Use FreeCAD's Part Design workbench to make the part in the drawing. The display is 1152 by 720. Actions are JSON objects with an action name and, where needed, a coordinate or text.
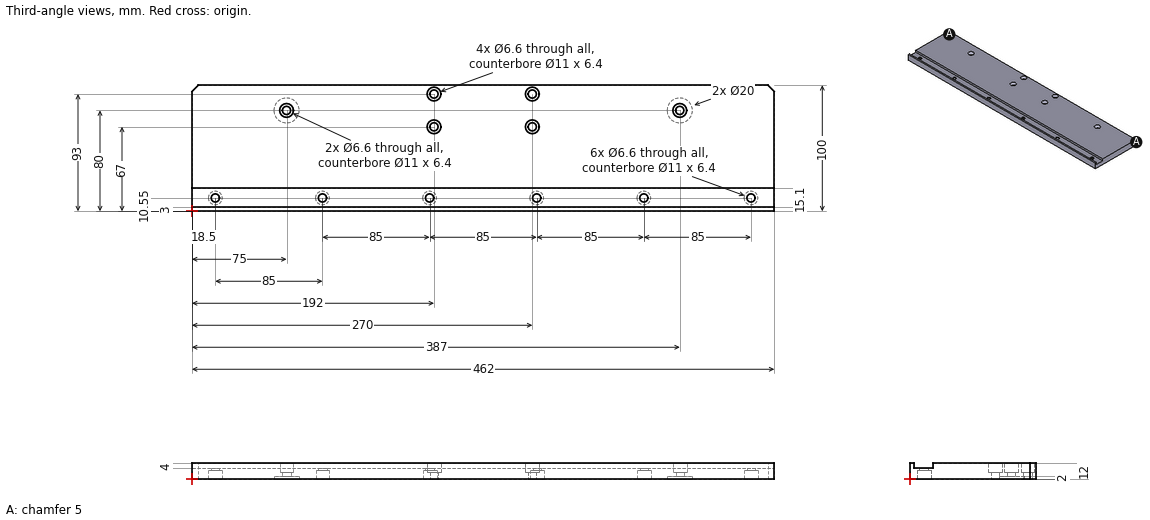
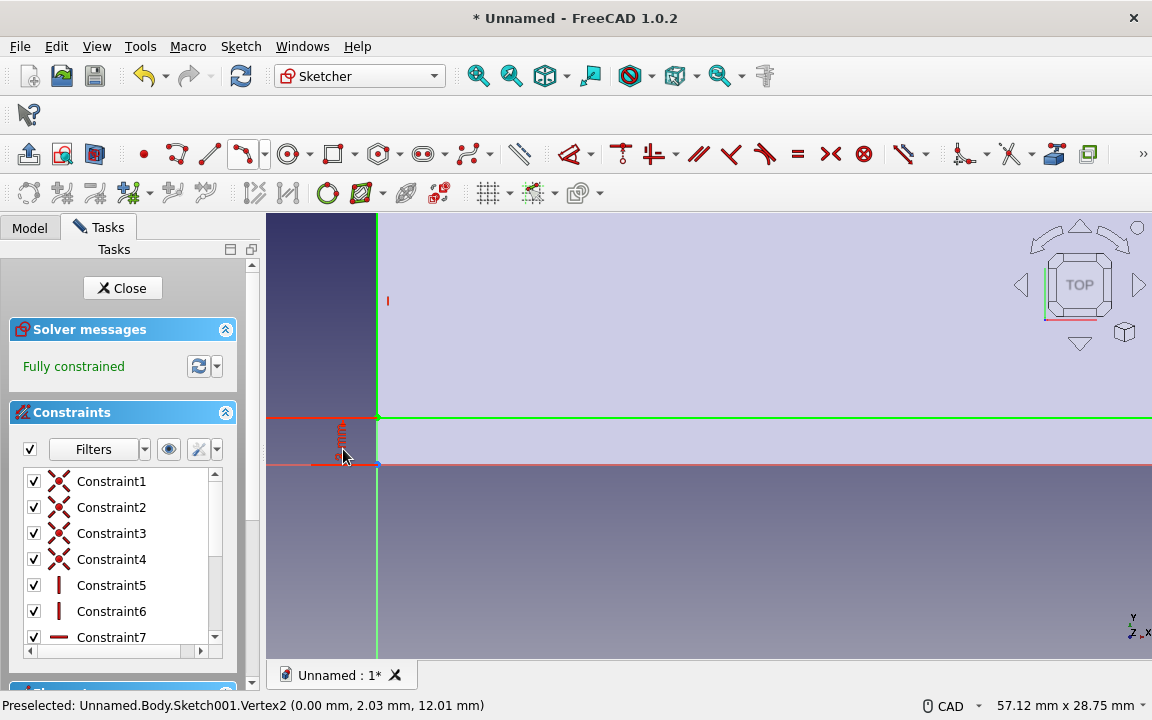
{"action": "left_click", "coordinate": [123, 288]}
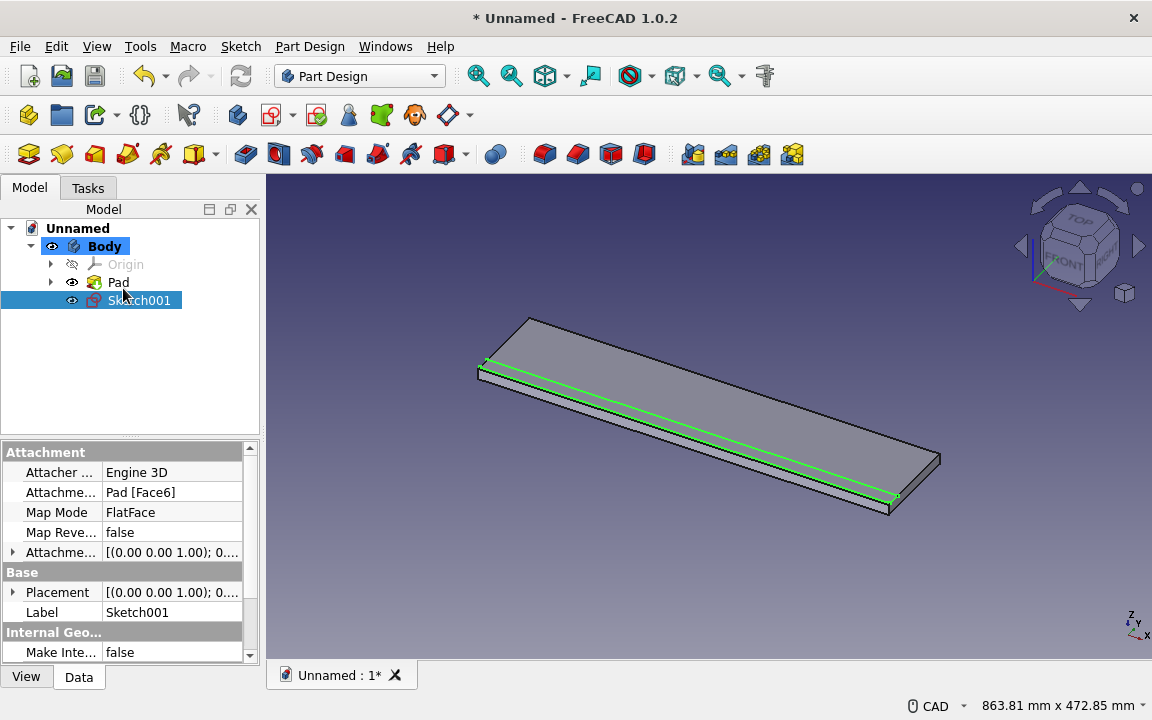
{"action": "left_click", "coordinate": [246, 154]}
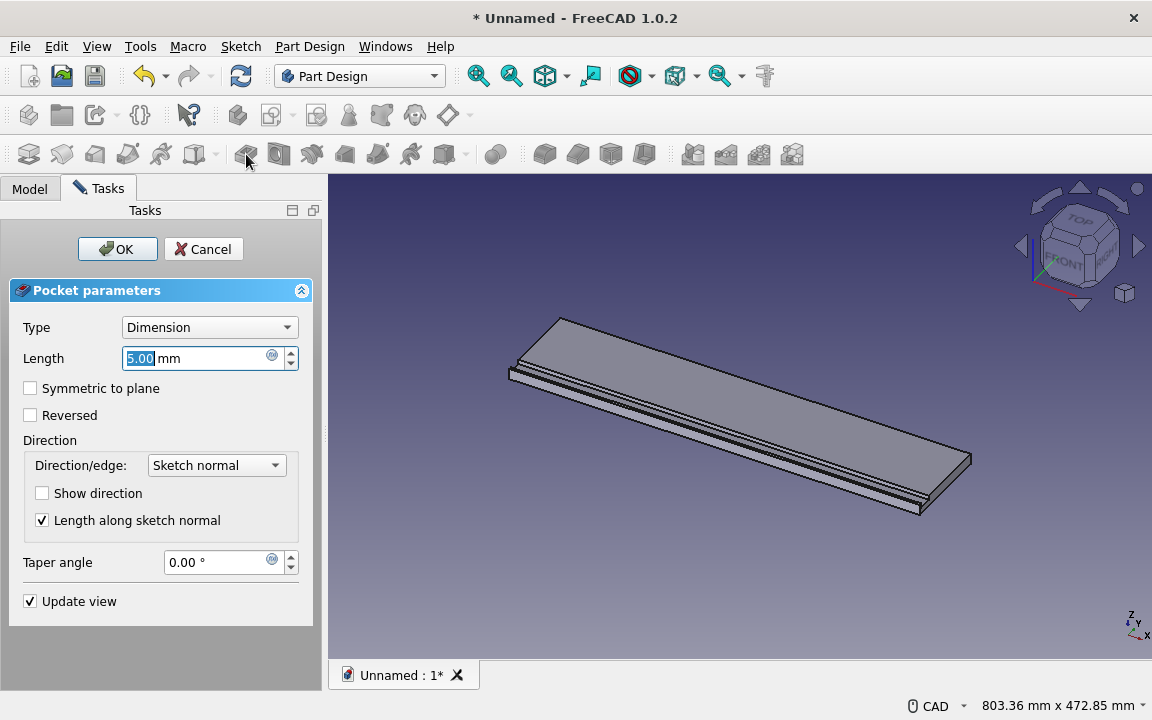
{"action": "type", "text": "4"}
{"action": "key", "text": "Tab"}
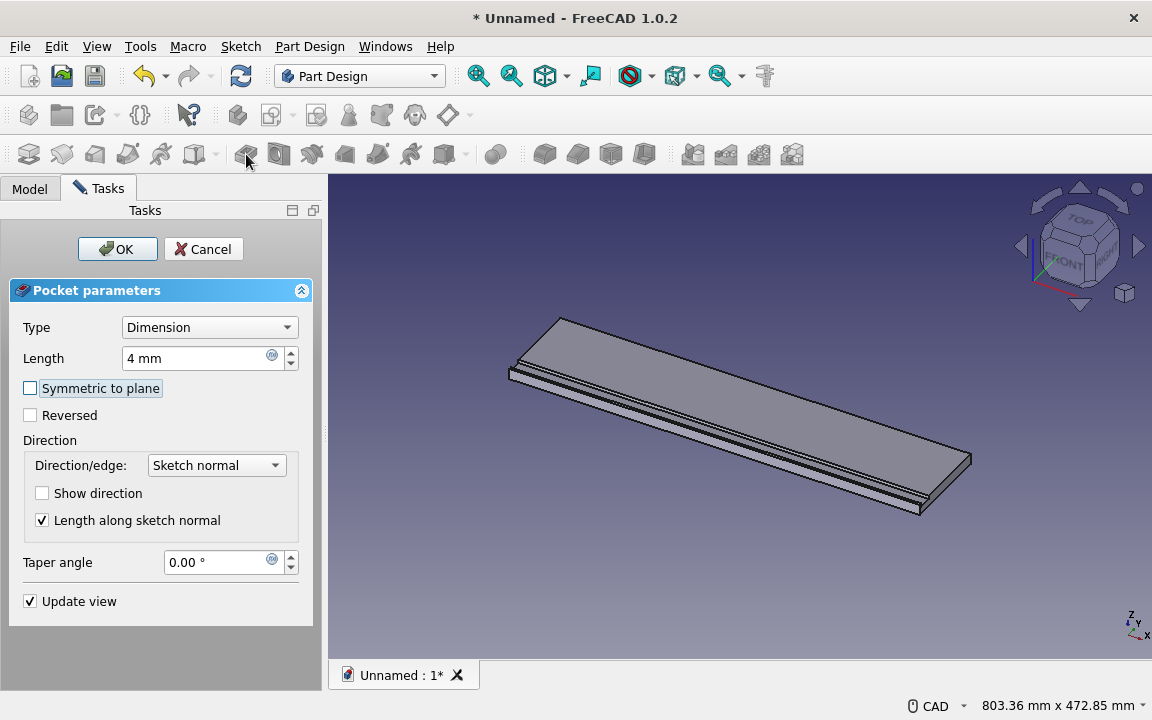
{"action": "left_click", "coordinate": [118, 249]}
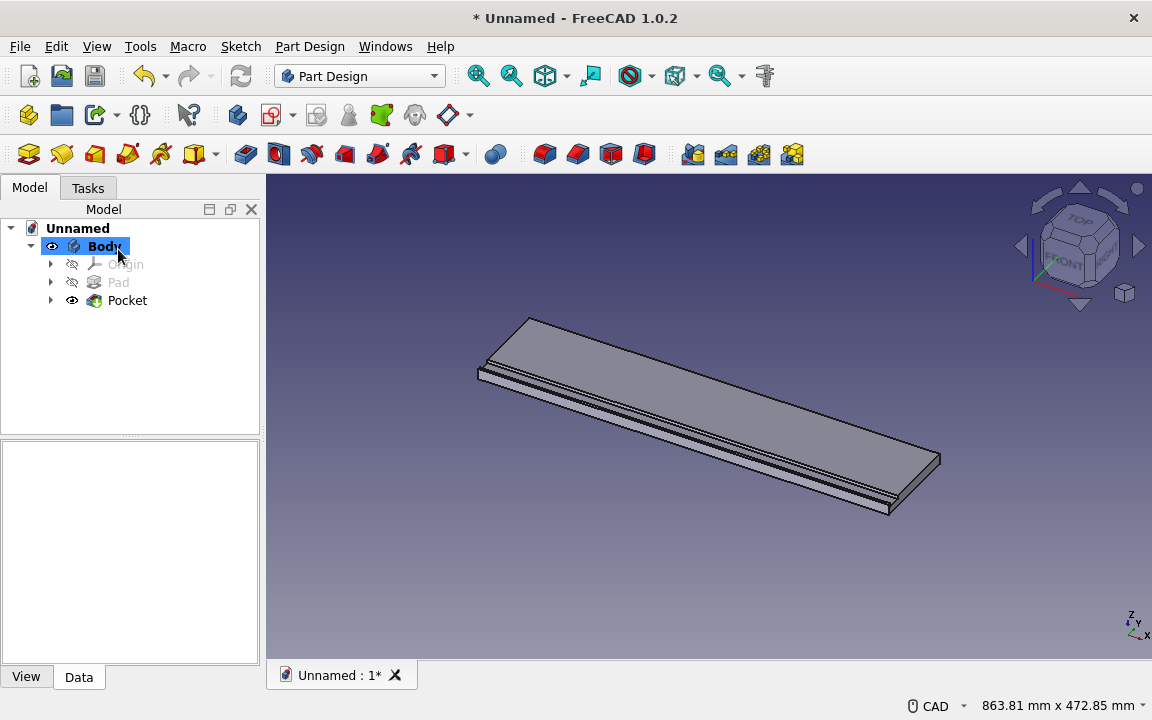
{"action": "left_click", "coordinate": [831, 445]}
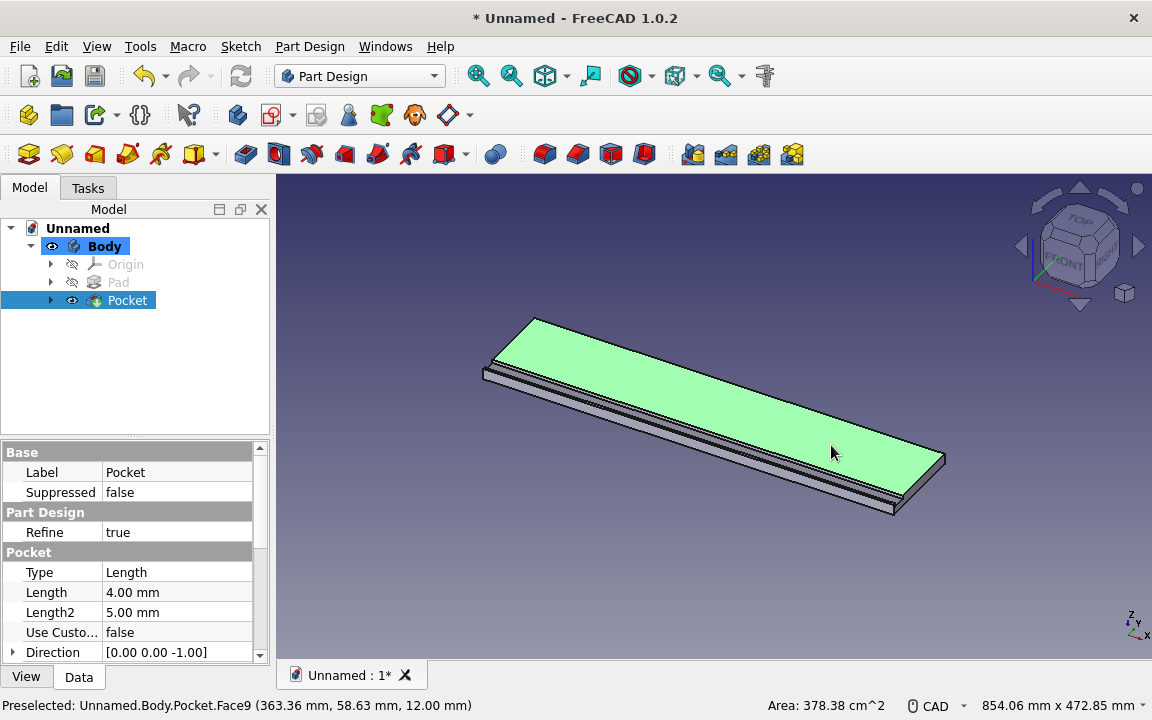
{"action": "left_click", "coordinate": [270, 116]}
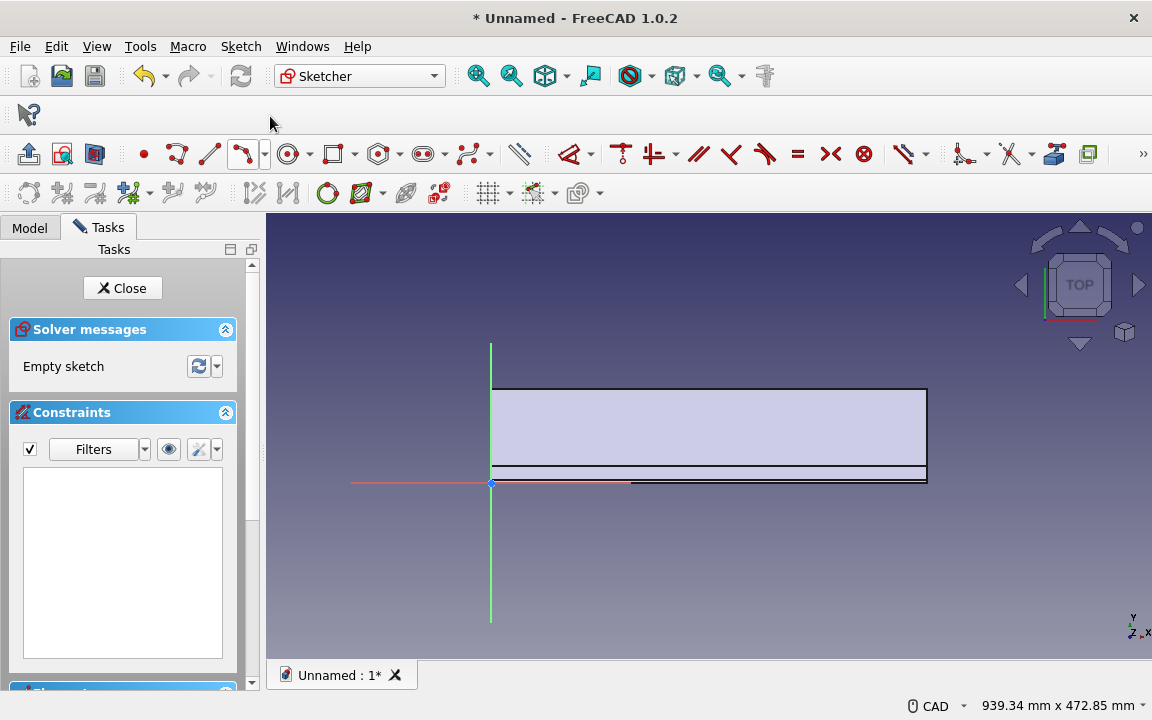
{"action": "scroll", "coordinate": [723, 402], "scroll_direction": "up", "scroll_amount": 9}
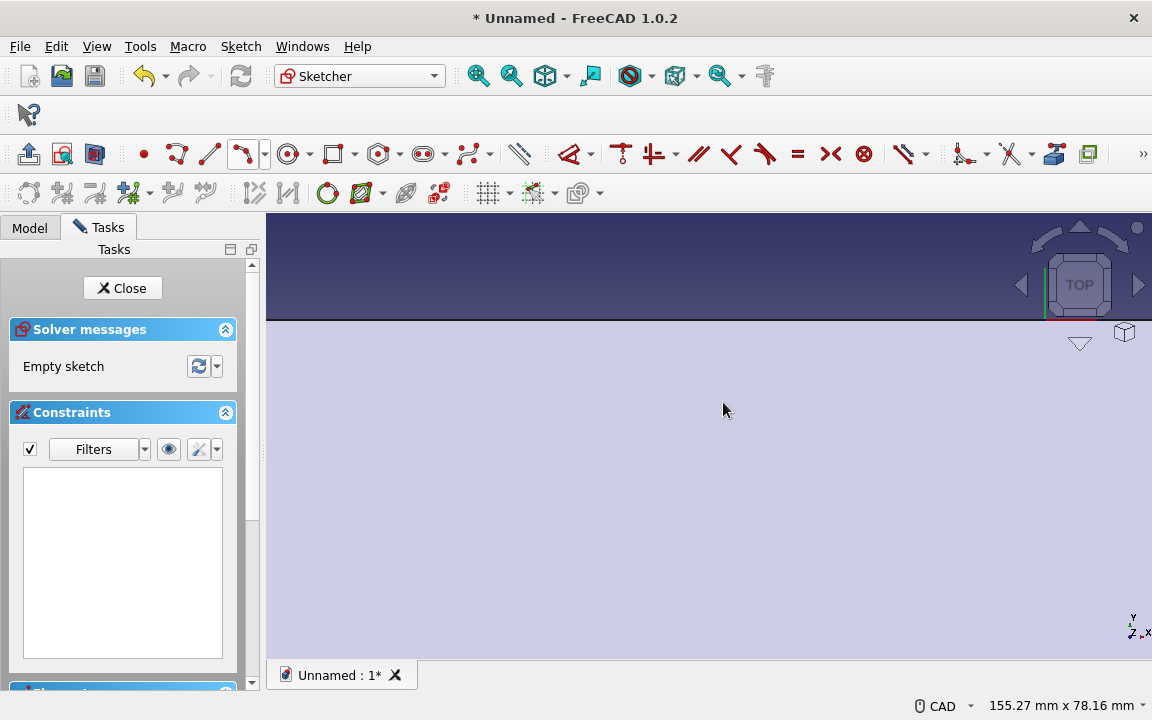
{"action": "left_click", "coordinate": [288, 154]}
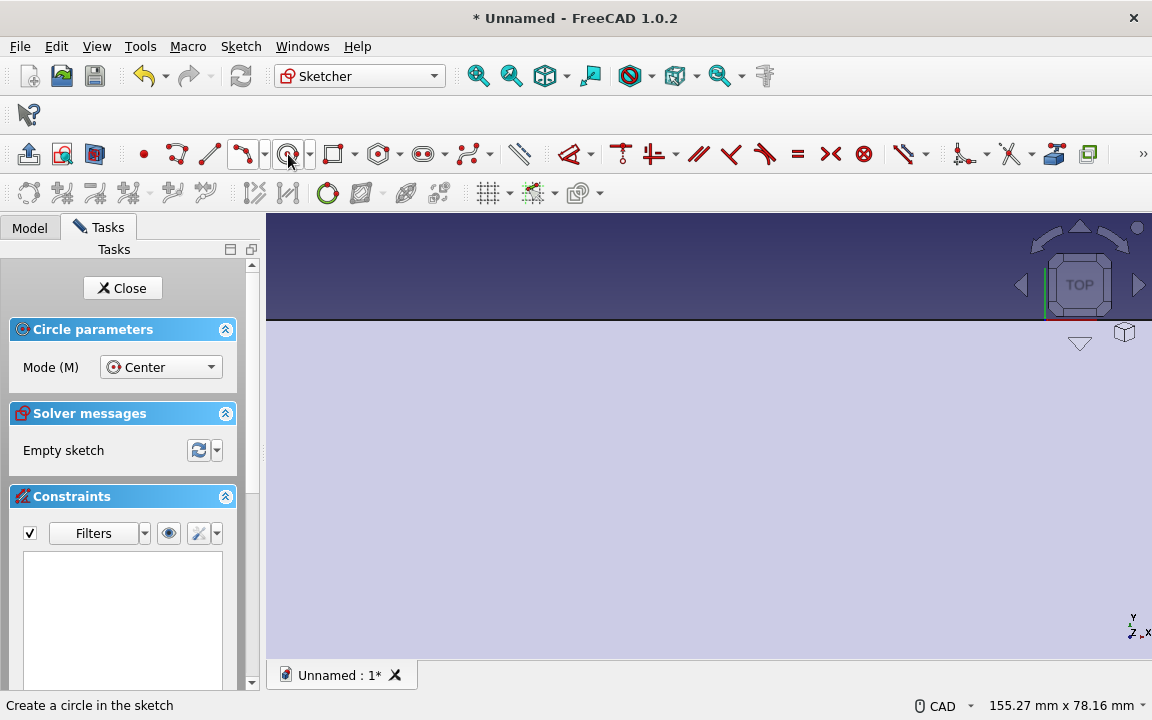
{"action": "left_click", "coordinate": [413, 360]}
{"action": "mouse_move", "coordinate": [426, 347]}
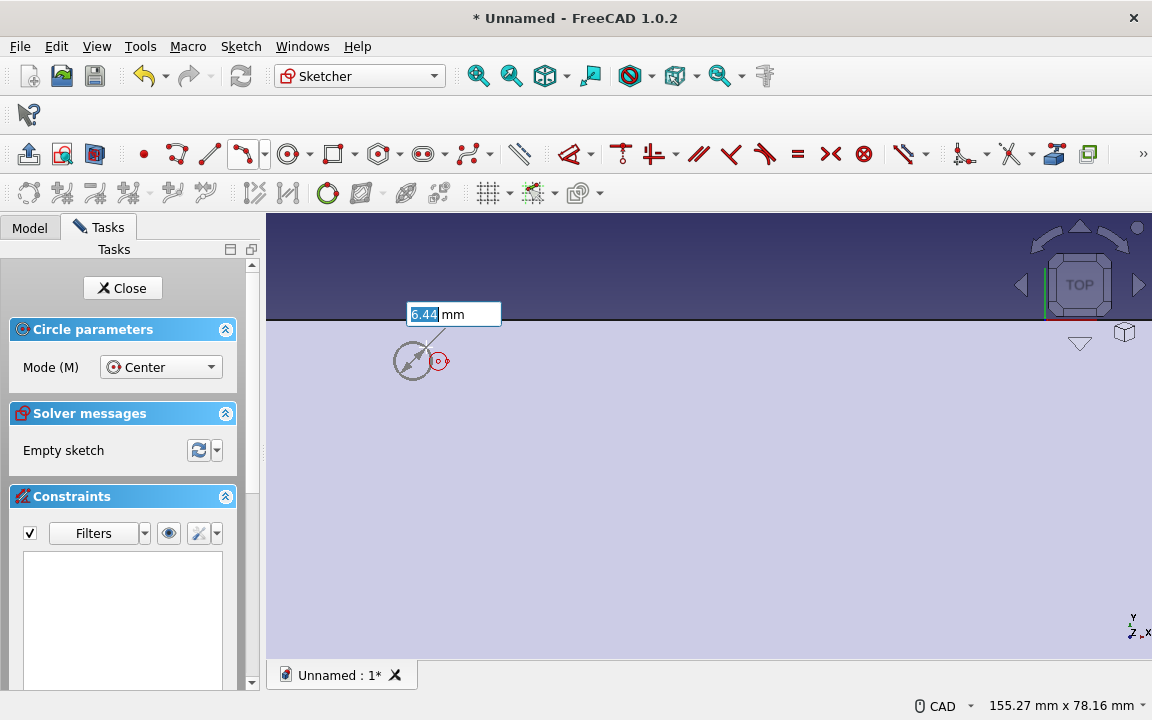
{"action": "type", "text": "6.6"}
{"action": "key", "text": "Return"}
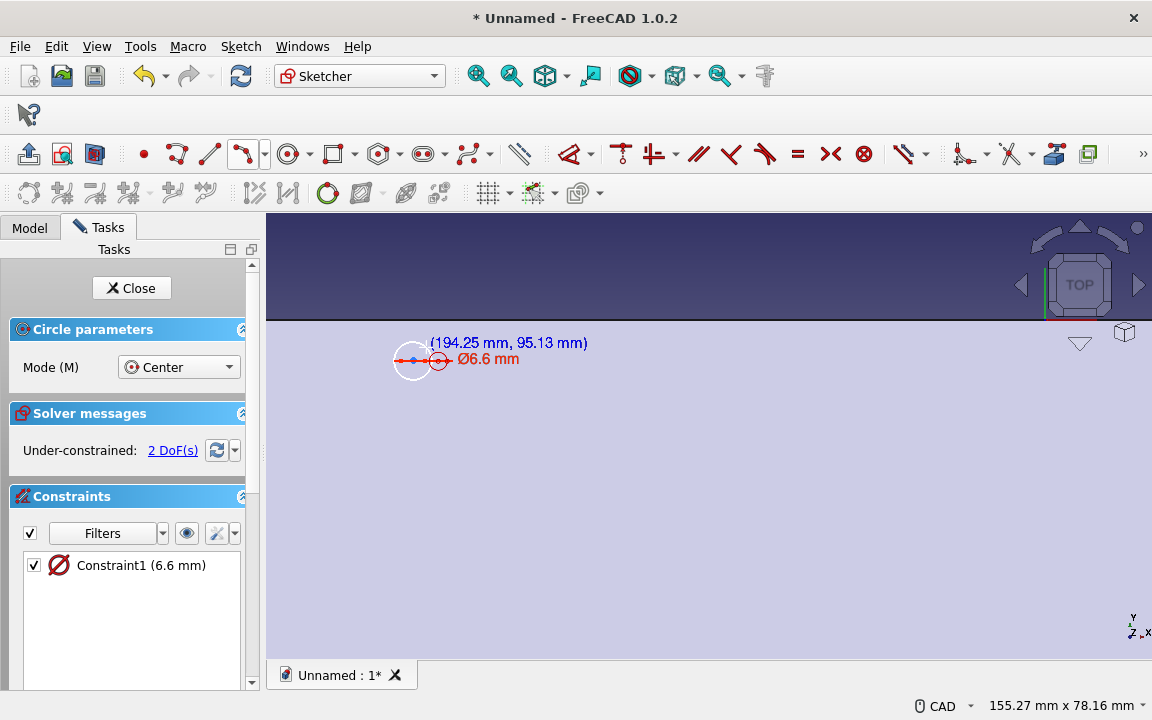
{"action": "left_click", "coordinate": [858, 360]}
{"action": "mouse_move", "coordinate": [872, 347]}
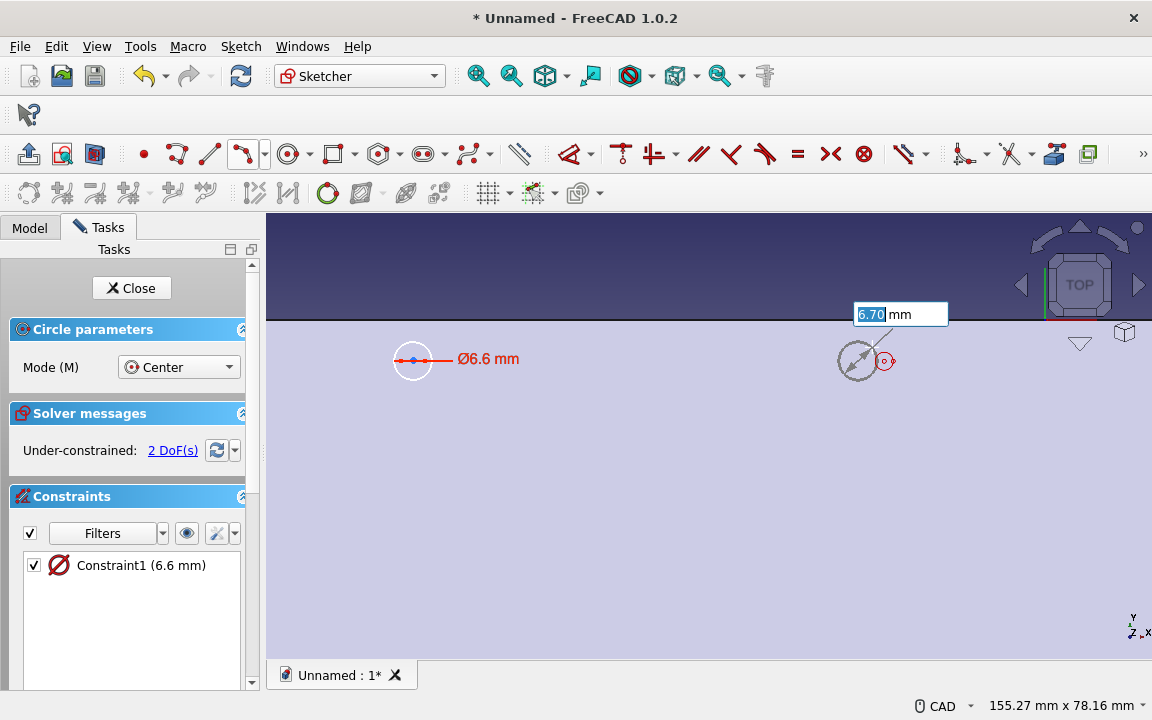
{"action": "type", "text": "6.6"}
{"action": "key", "text": "Return"}